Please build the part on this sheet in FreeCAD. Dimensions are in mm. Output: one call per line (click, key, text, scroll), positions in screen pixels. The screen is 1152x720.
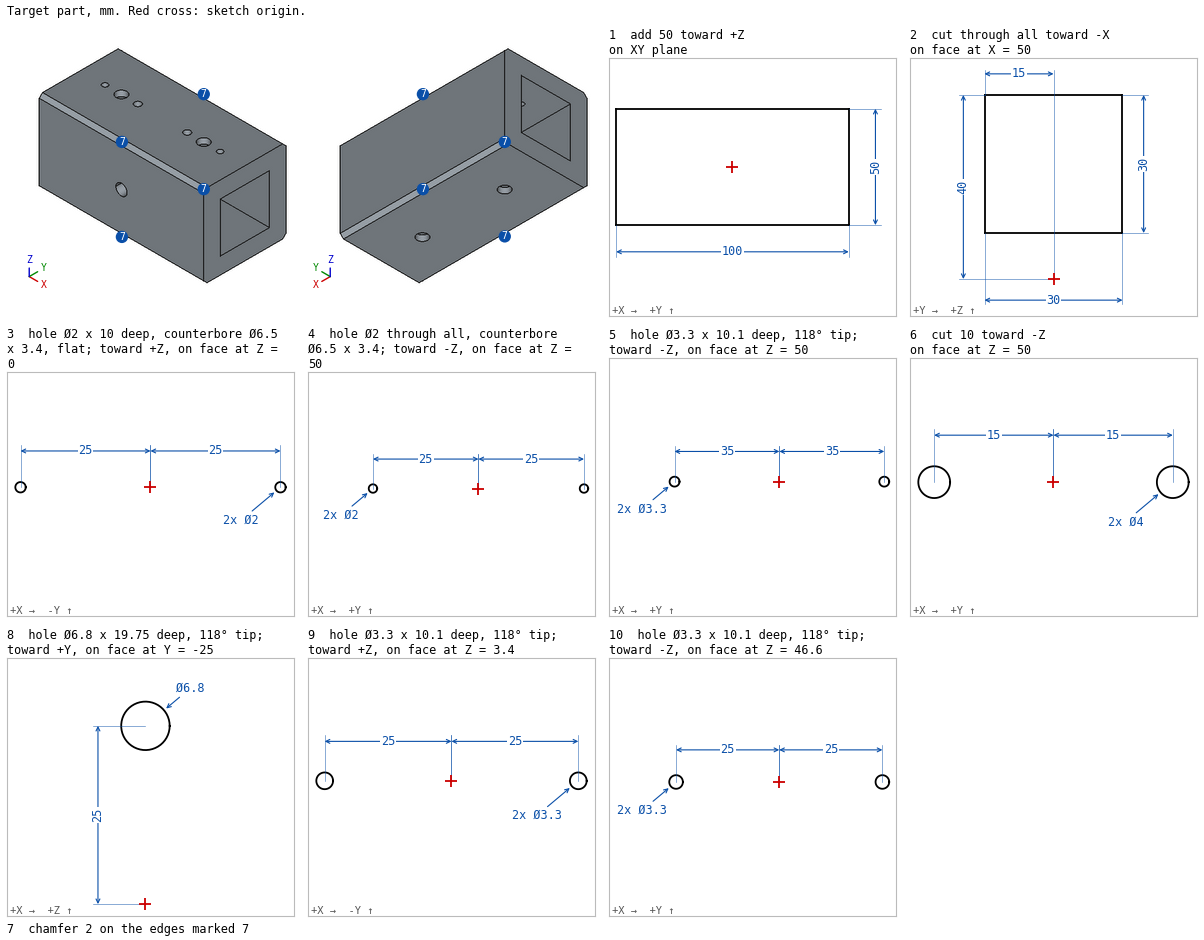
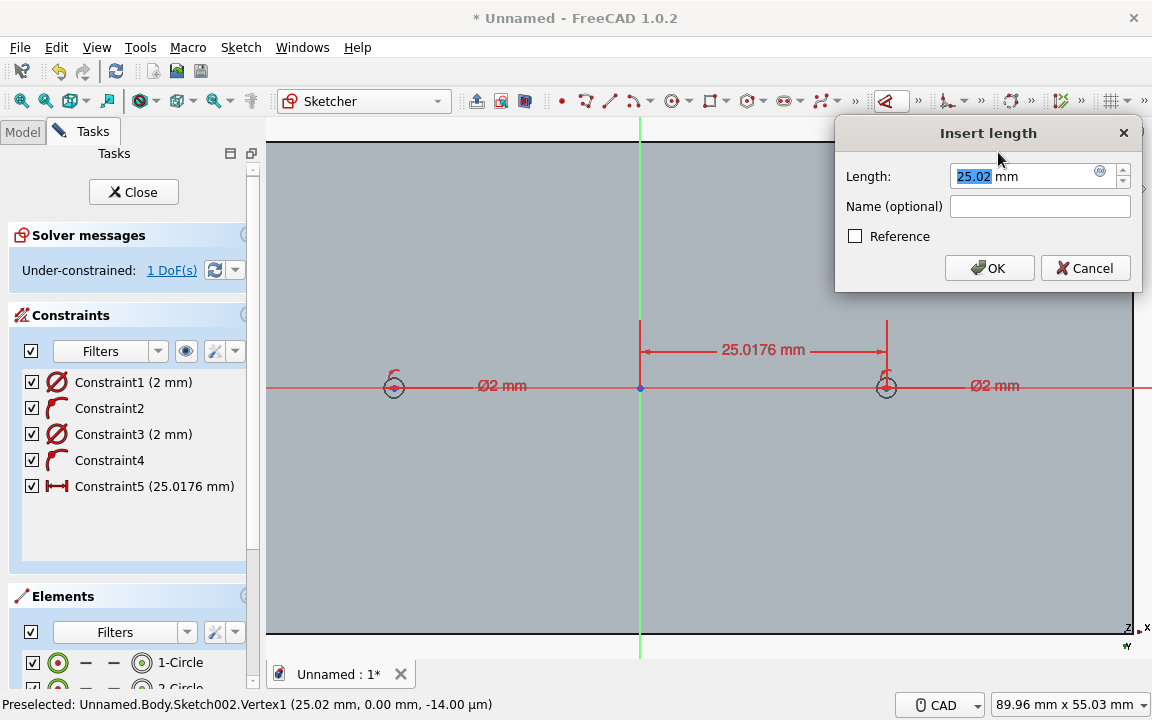
text(25)
key(Return)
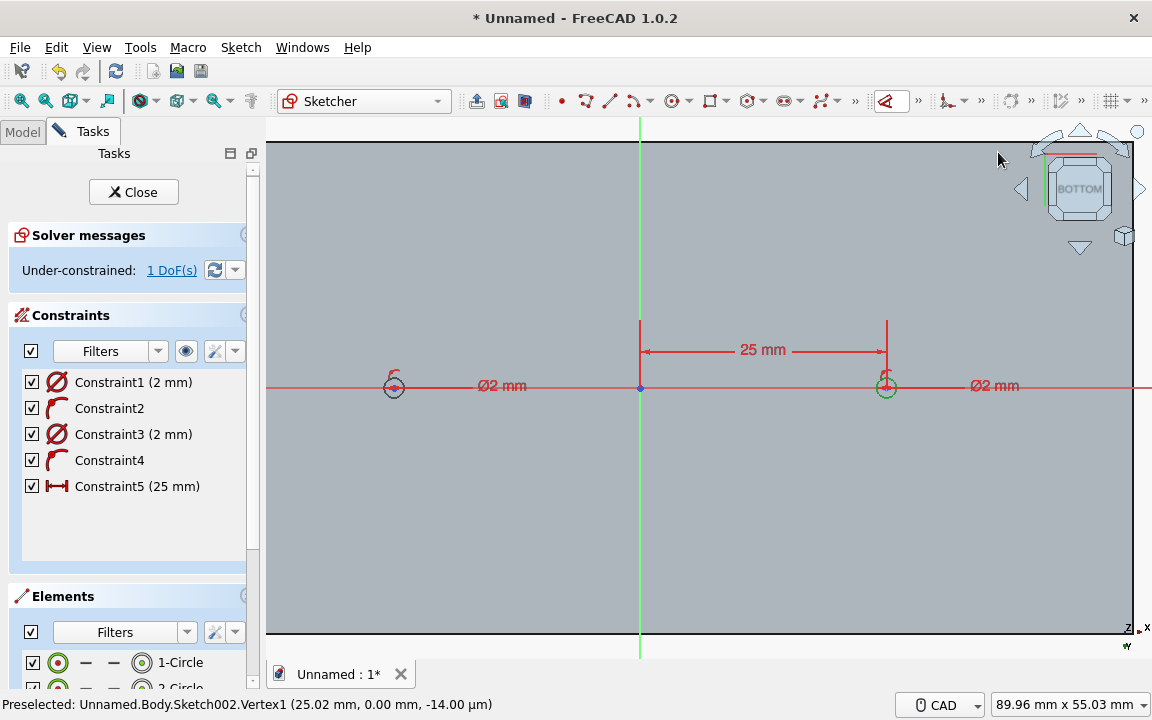
click(394, 388)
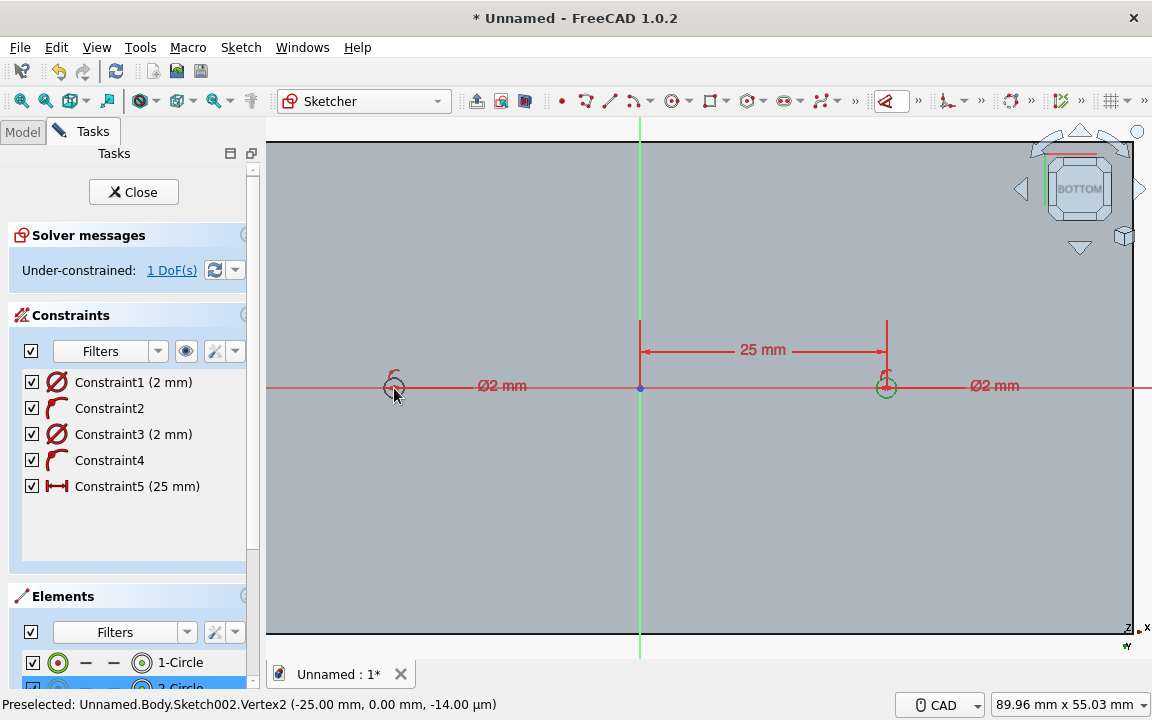
key(l)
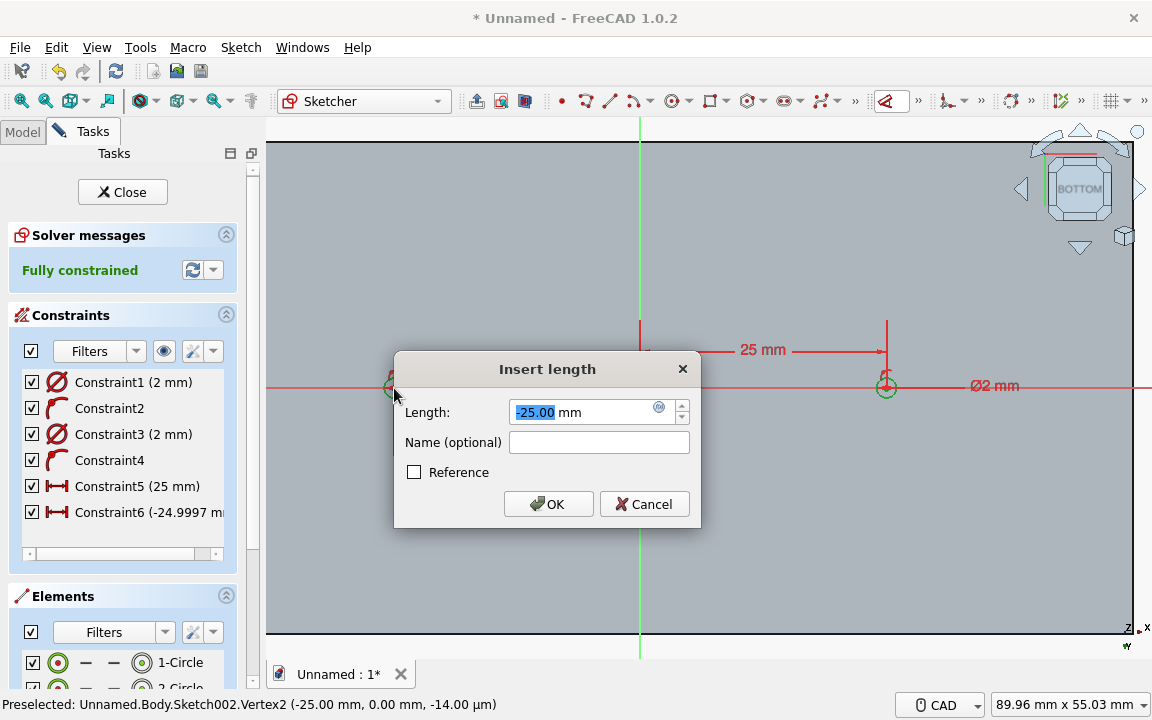
text(-25)
key(Return)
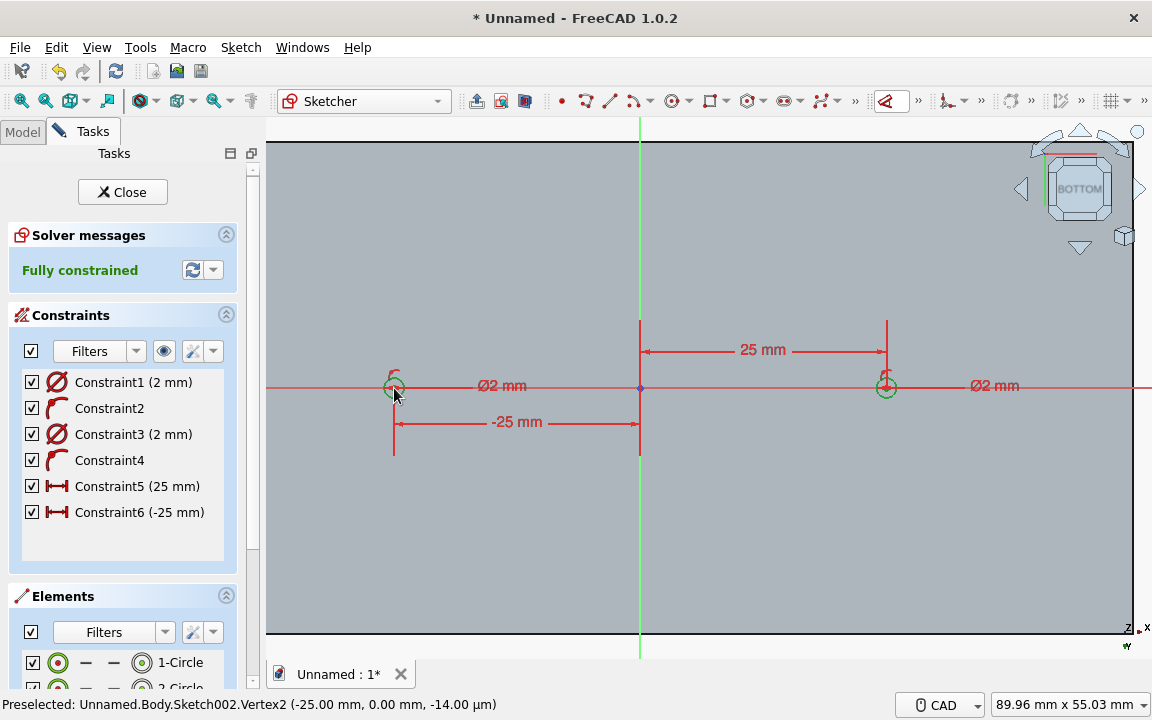
click(123, 192)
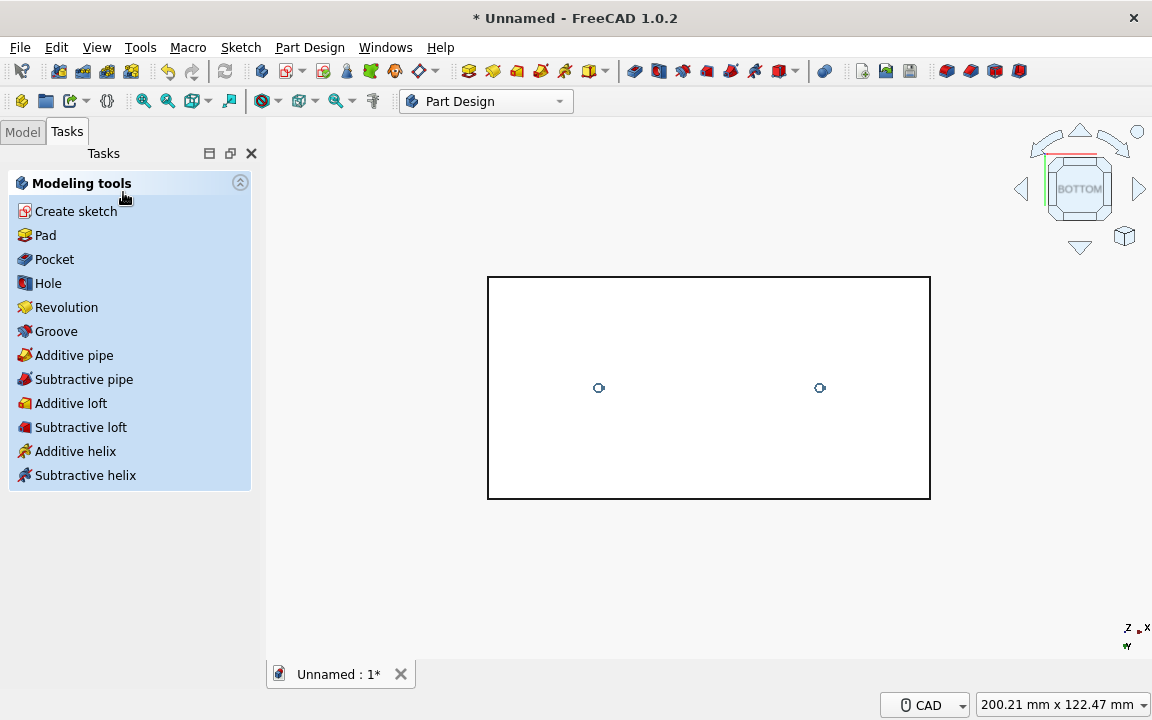
click(660, 72)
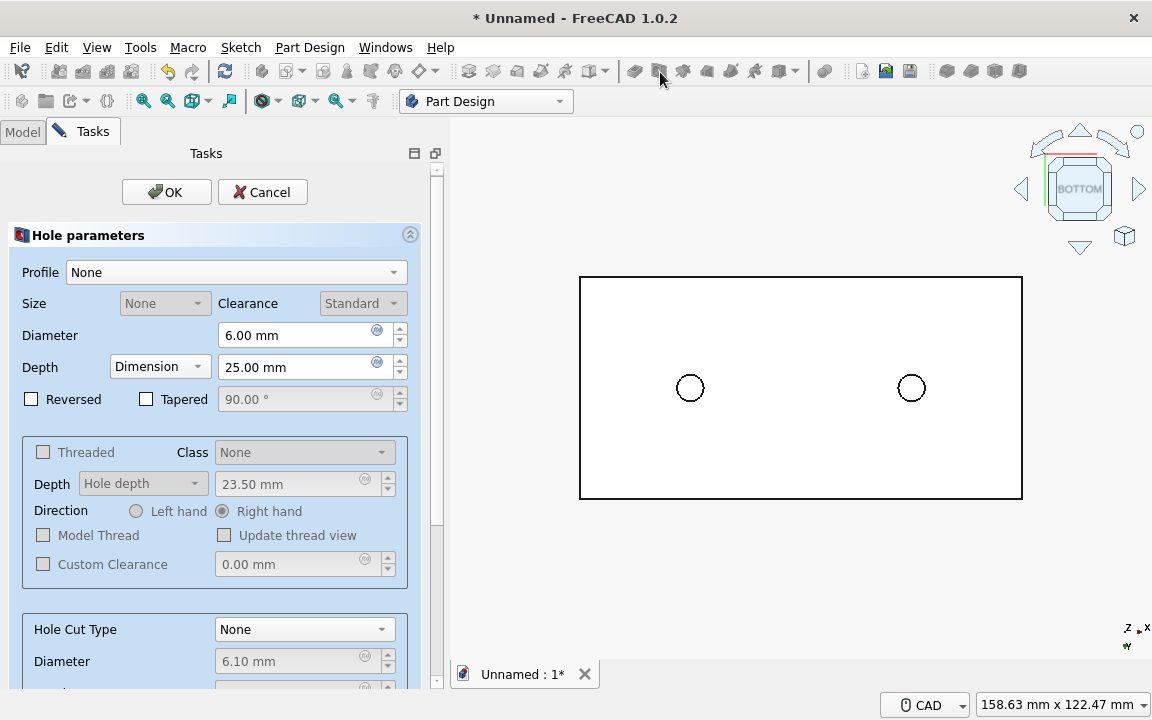
triple_click(305, 335)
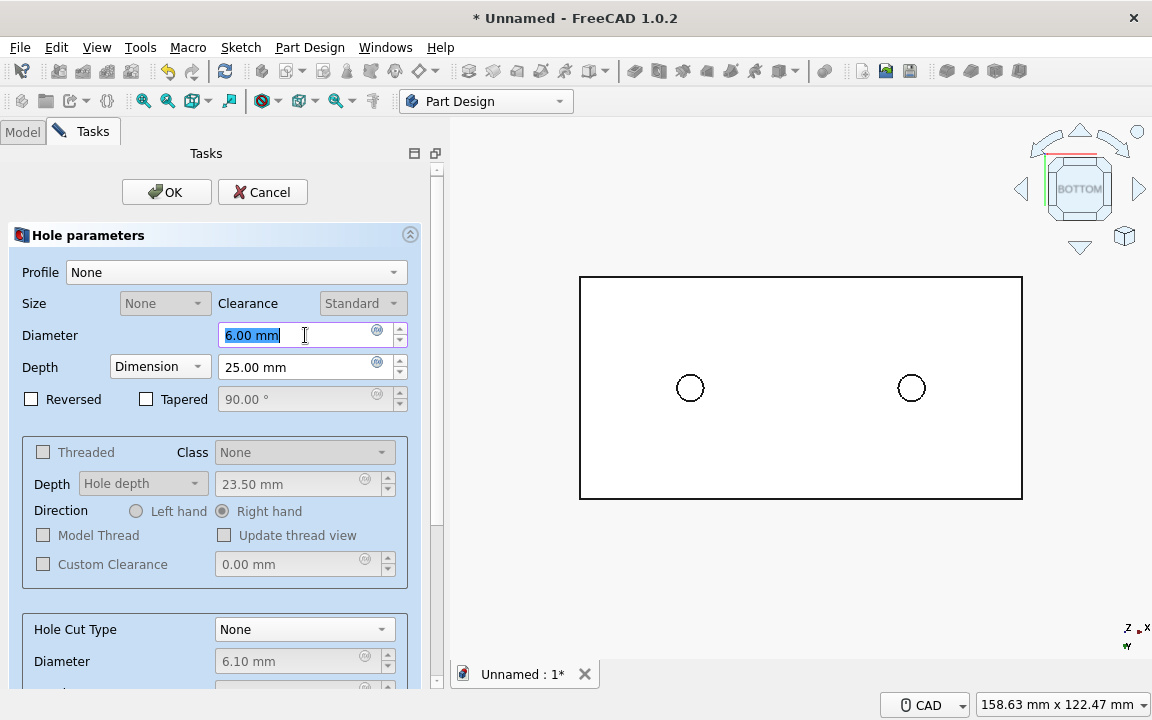
text(2)
key(Tab)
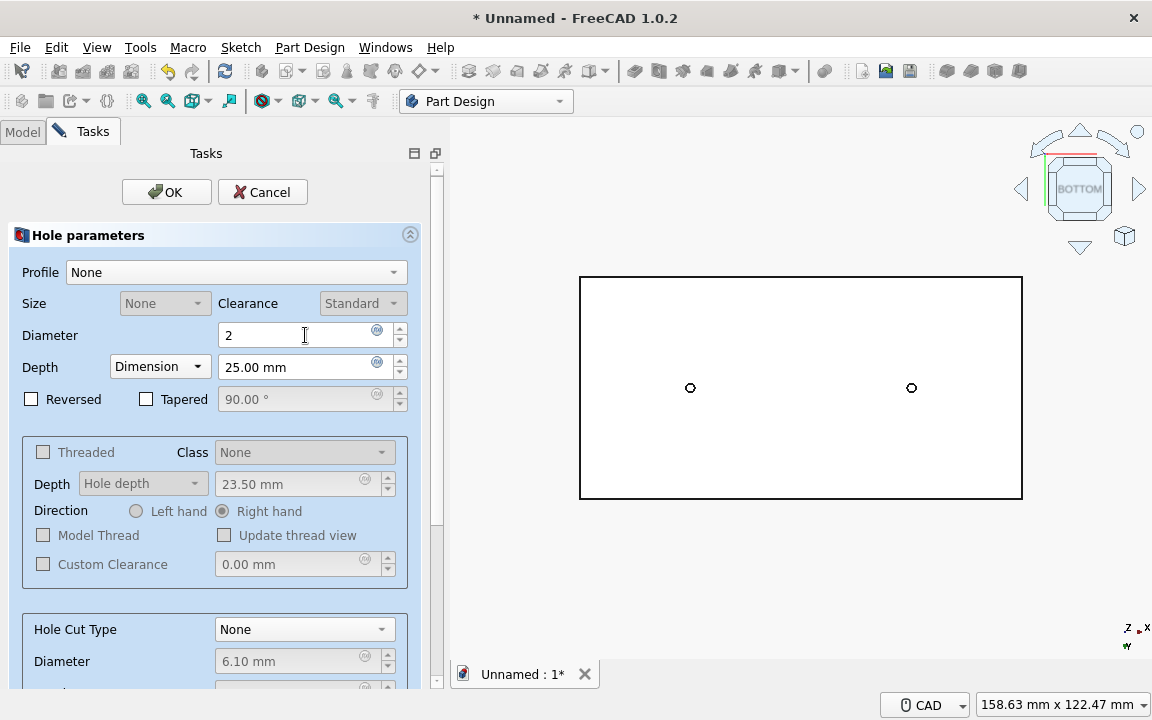
triple_click(305, 367)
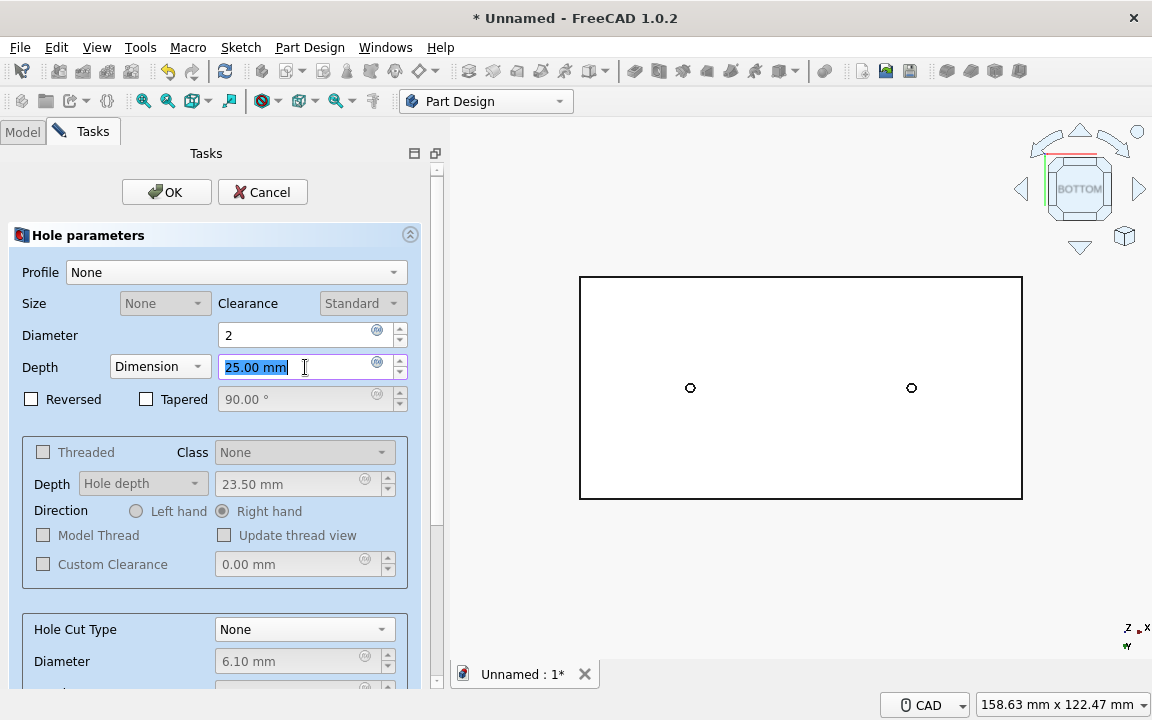
text(10)
key(Tab)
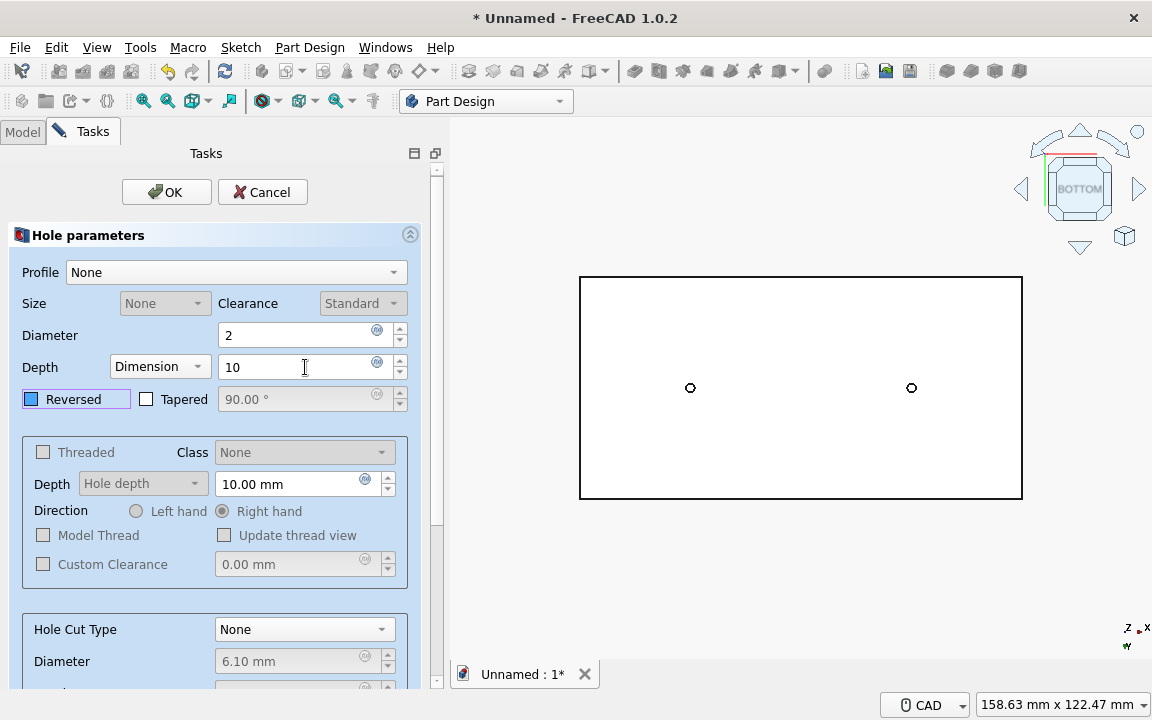
click(306, 630)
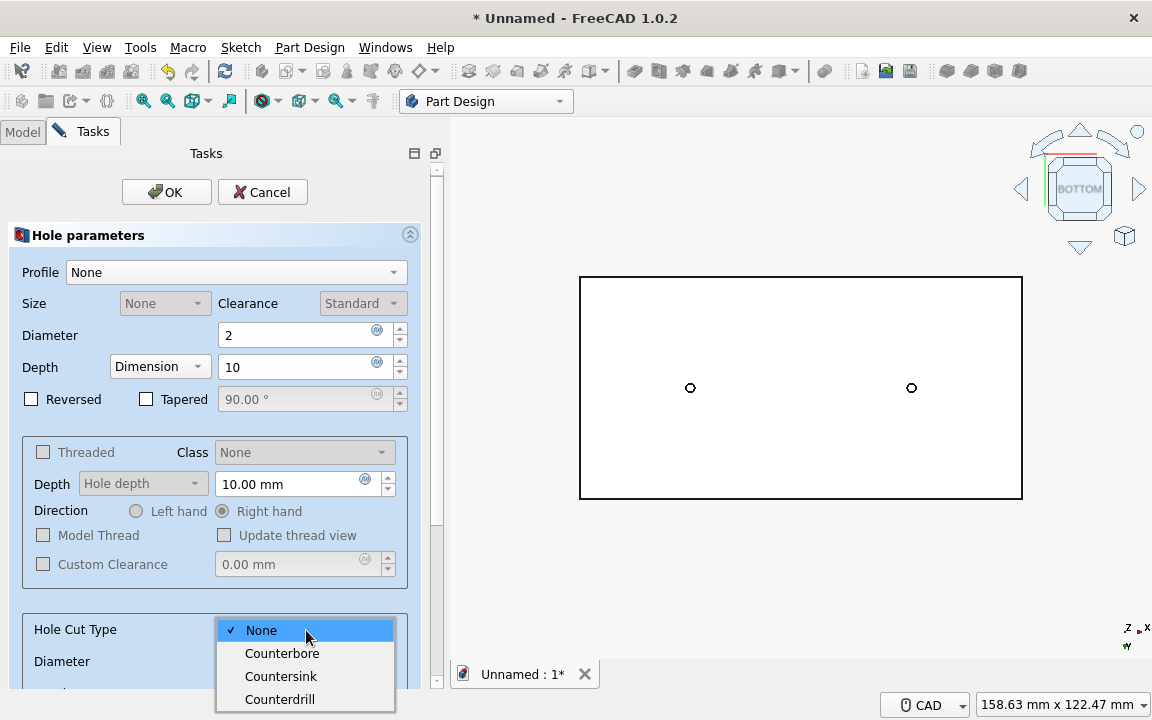
click(304, 654)